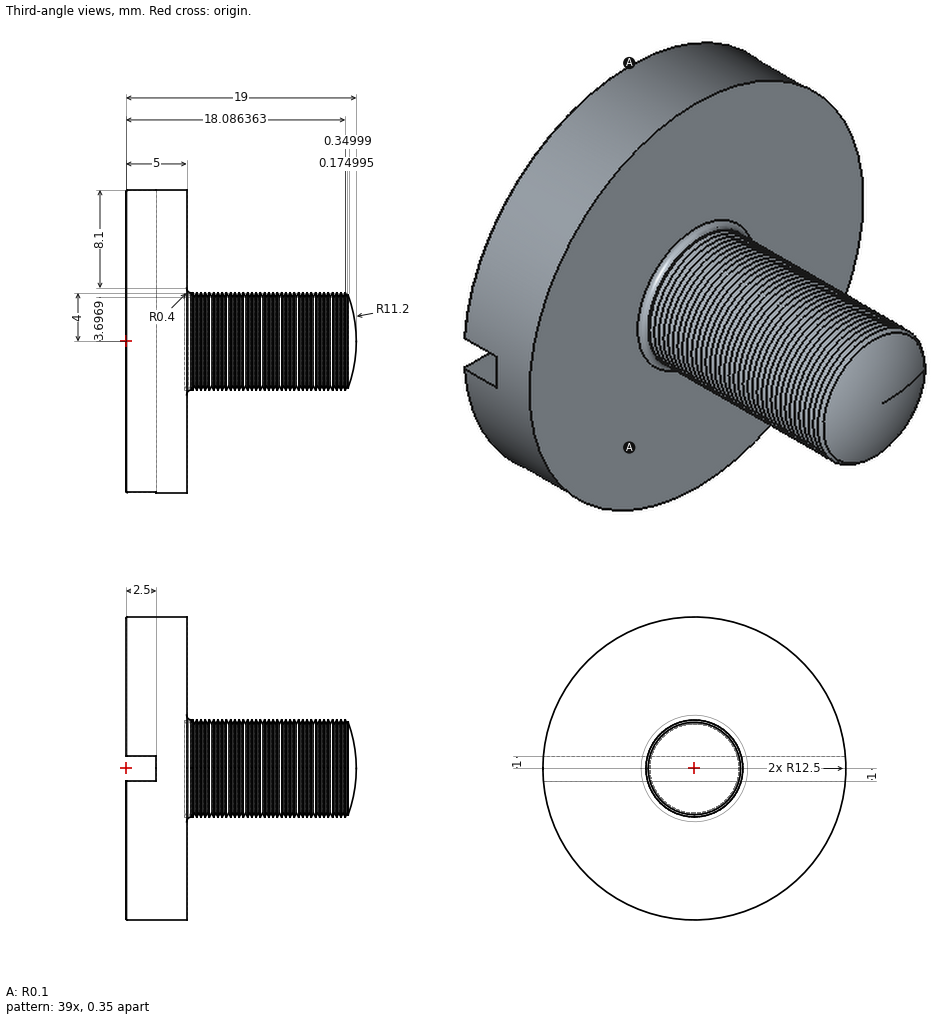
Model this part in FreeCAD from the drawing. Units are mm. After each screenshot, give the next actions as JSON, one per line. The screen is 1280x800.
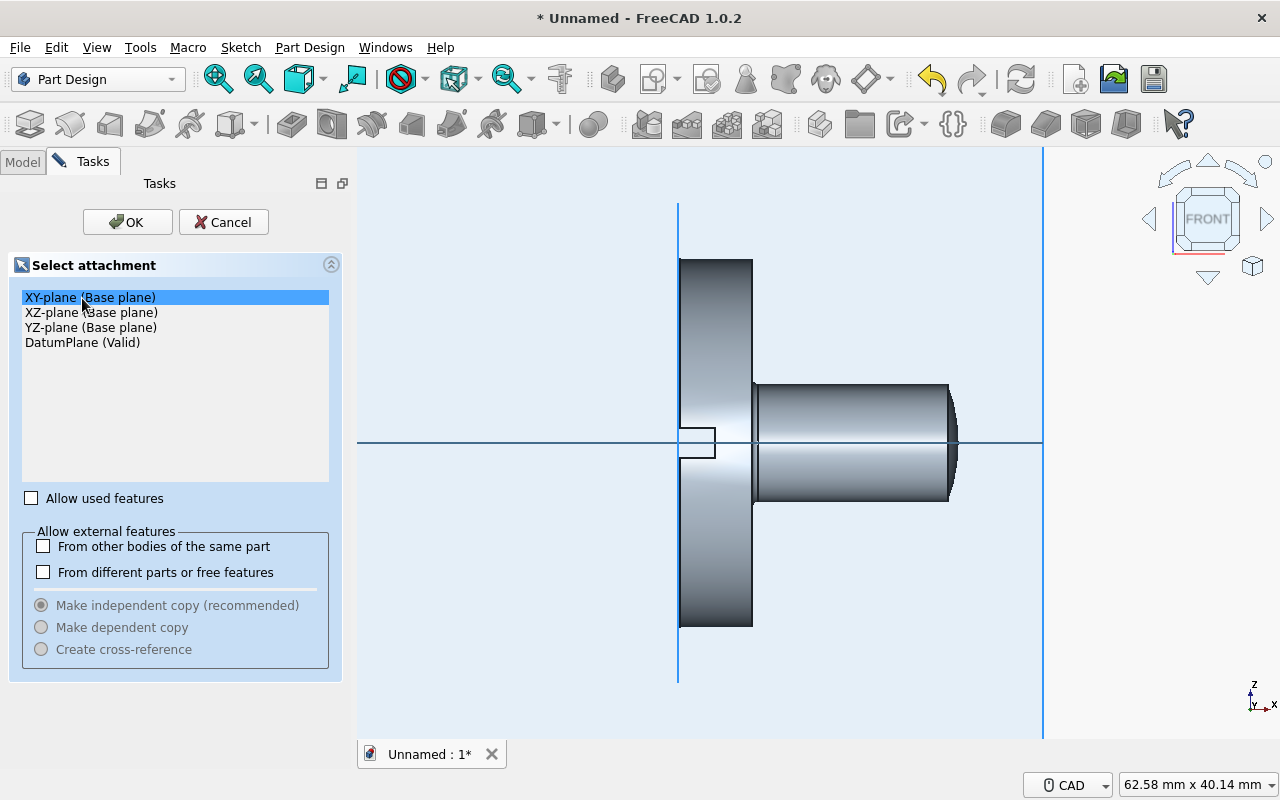
{"action": "left_click", "coordinate": [128, 222]}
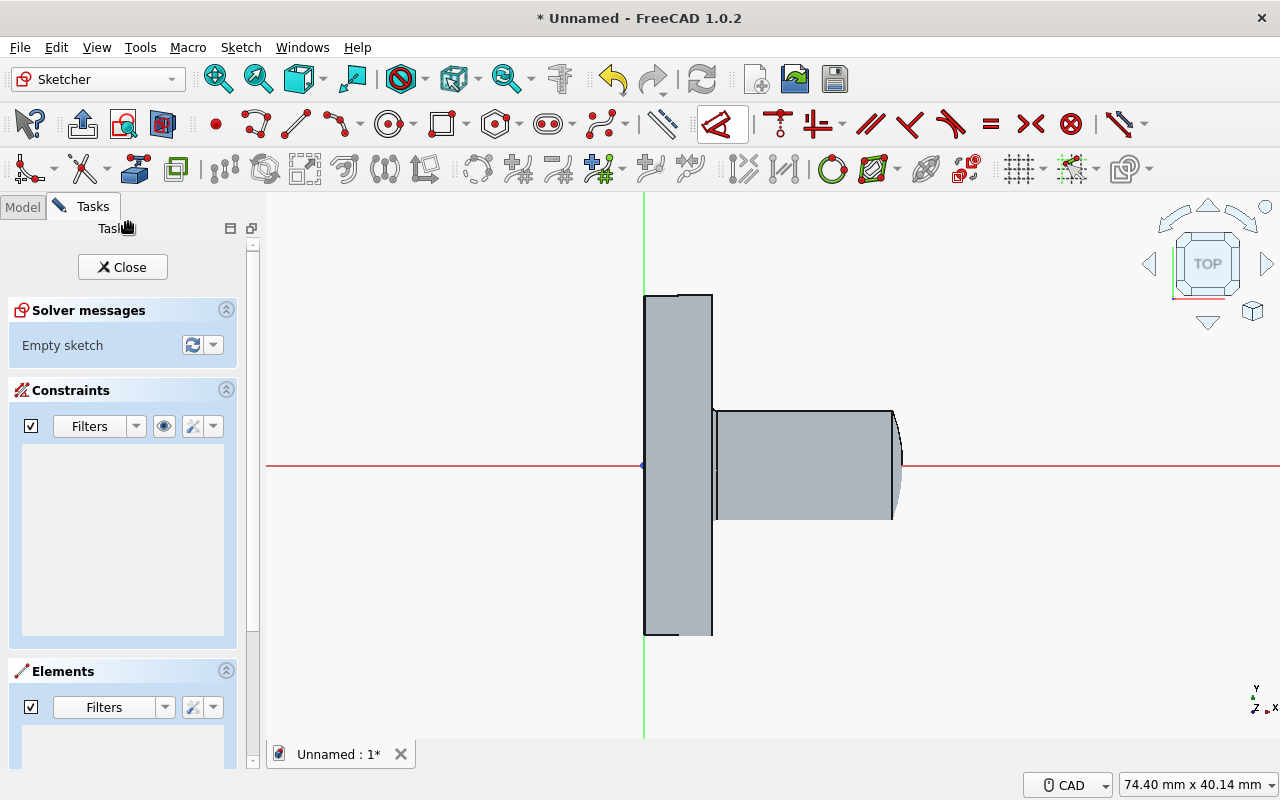
{"action": "left_click", "coordinate": [164, 124]}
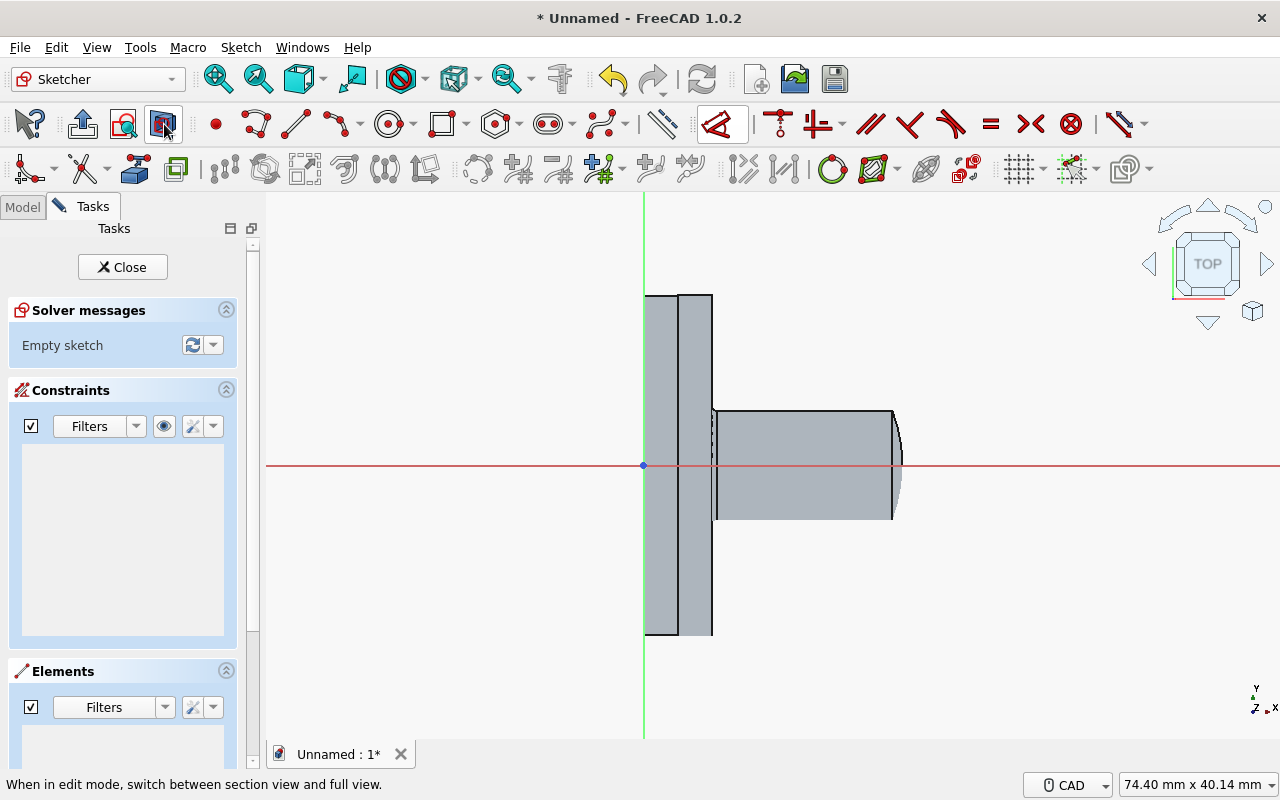
{"action": "scroll", "coordinate": [902, 410], "scroll_direction": "up", "scroll_amount": 15}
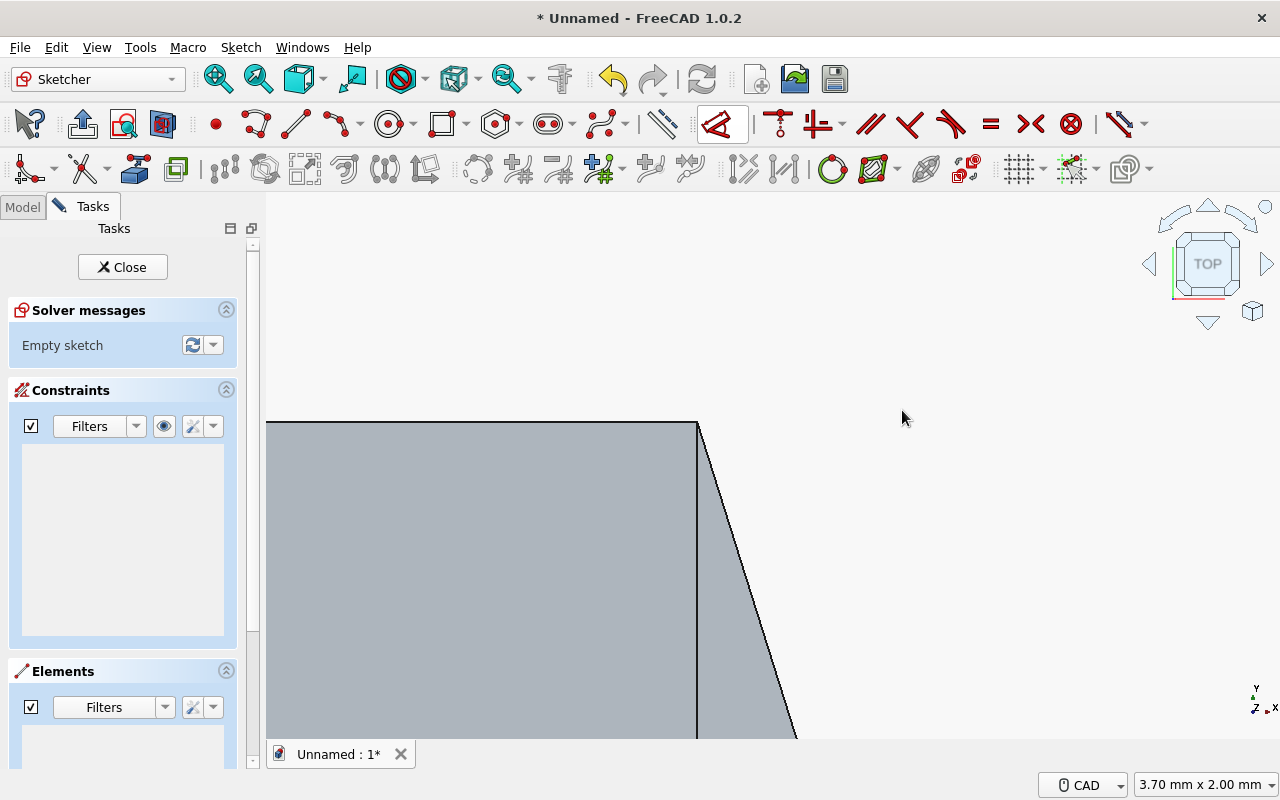
{"action": "scroll", "coordinate": [695, 463], "scroll_direction": "up", "scroll_amount": 7}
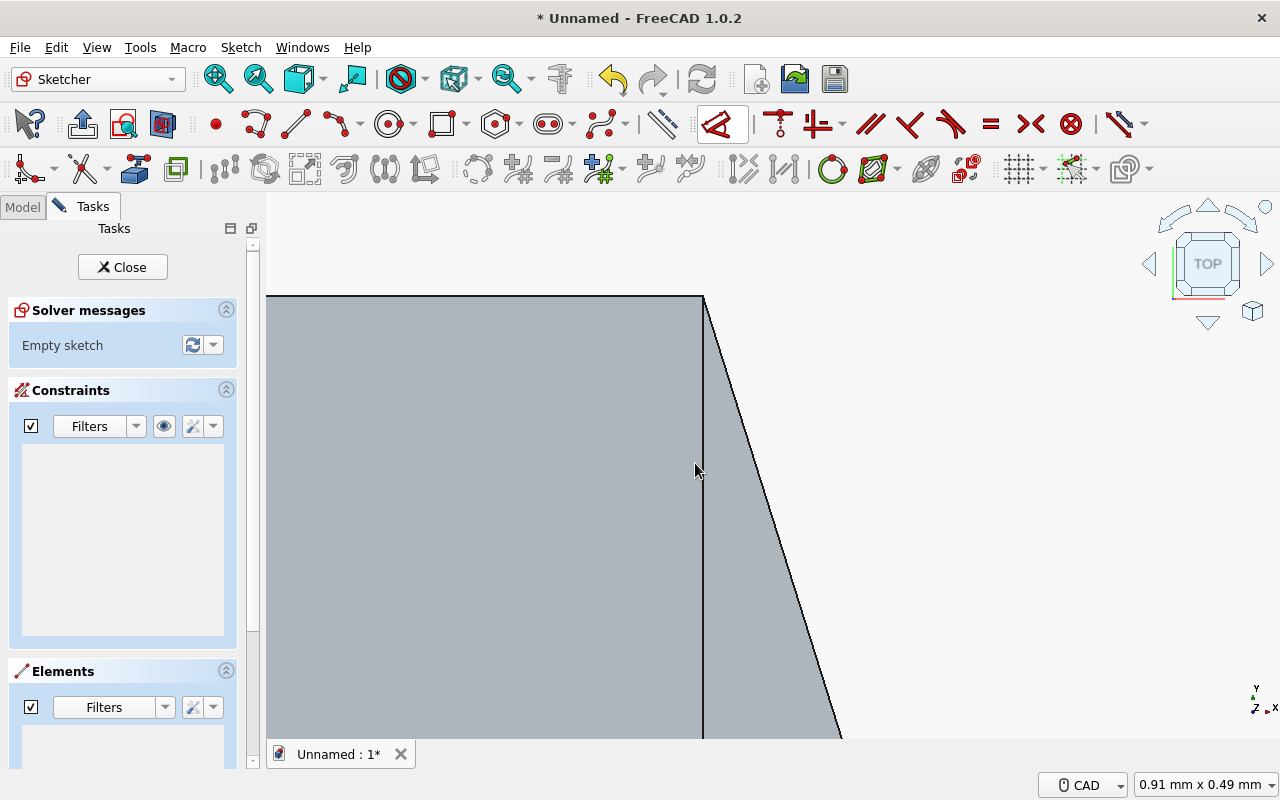
{"action": "left_click", "coordinate": [256, 124]}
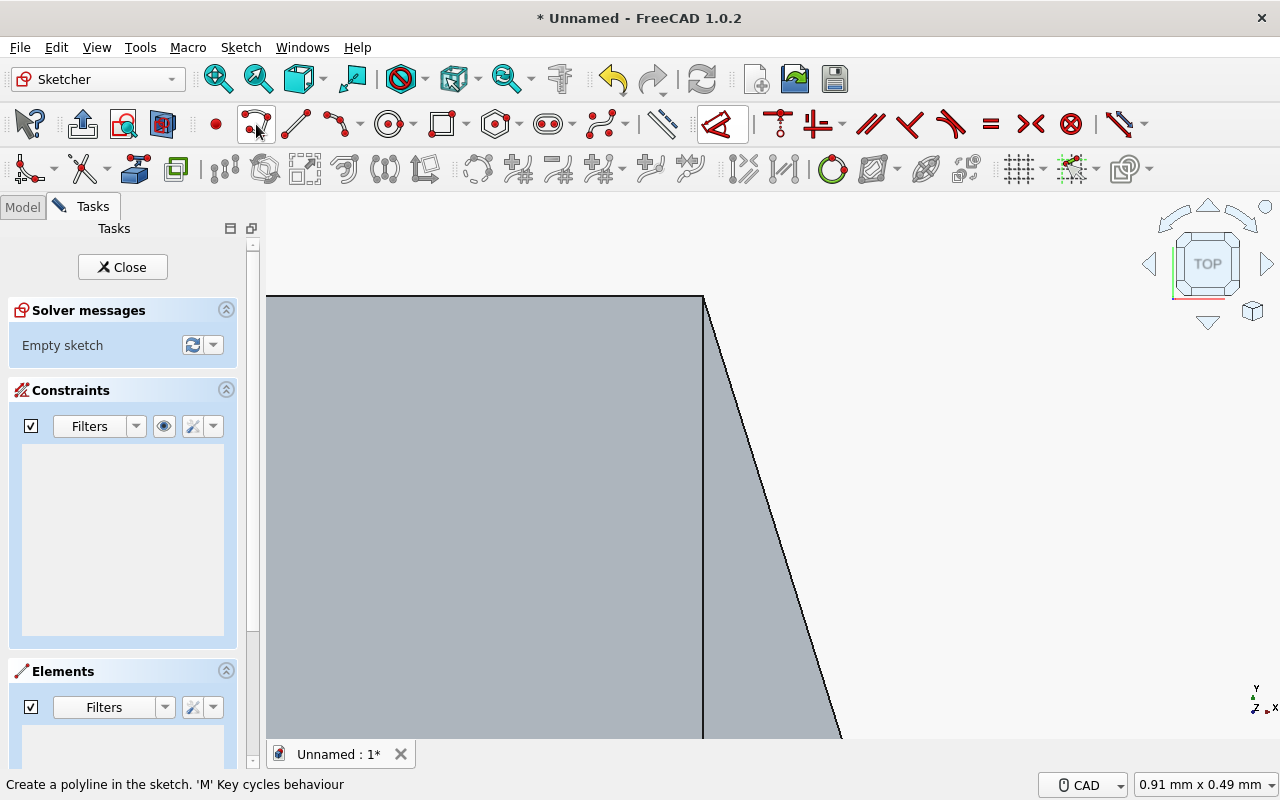
{"action": "left_click", "coordinate": [509, 296]}
{"action": "left_click", "coordinate": [703, 633]}
{"action": "left_click", "coordinate": [897, 296]}
{"action": "left_click", "coordinate": [509, 297]}
{"action": "key", "text": "Escape"}
{"action": "key", "text": "Escape"}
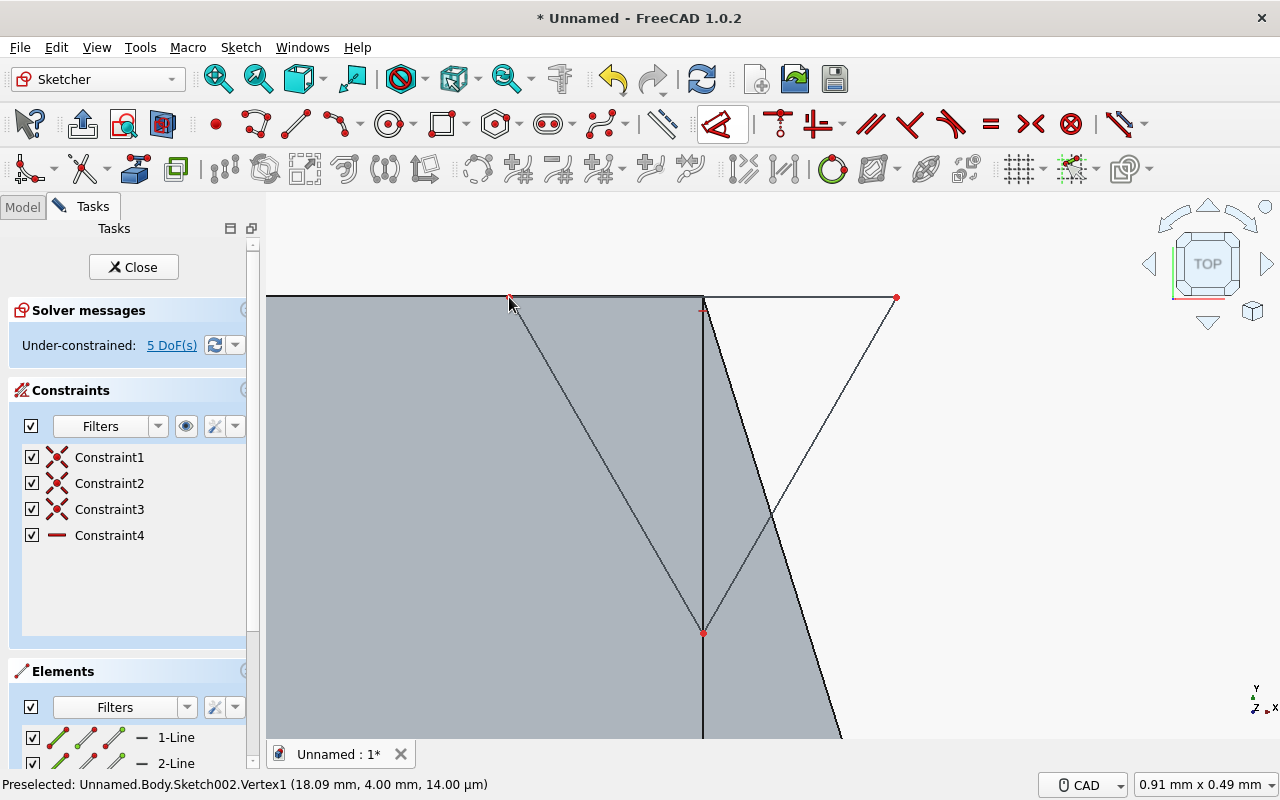
{"action": "left_click", "coordinate": [509, 297]}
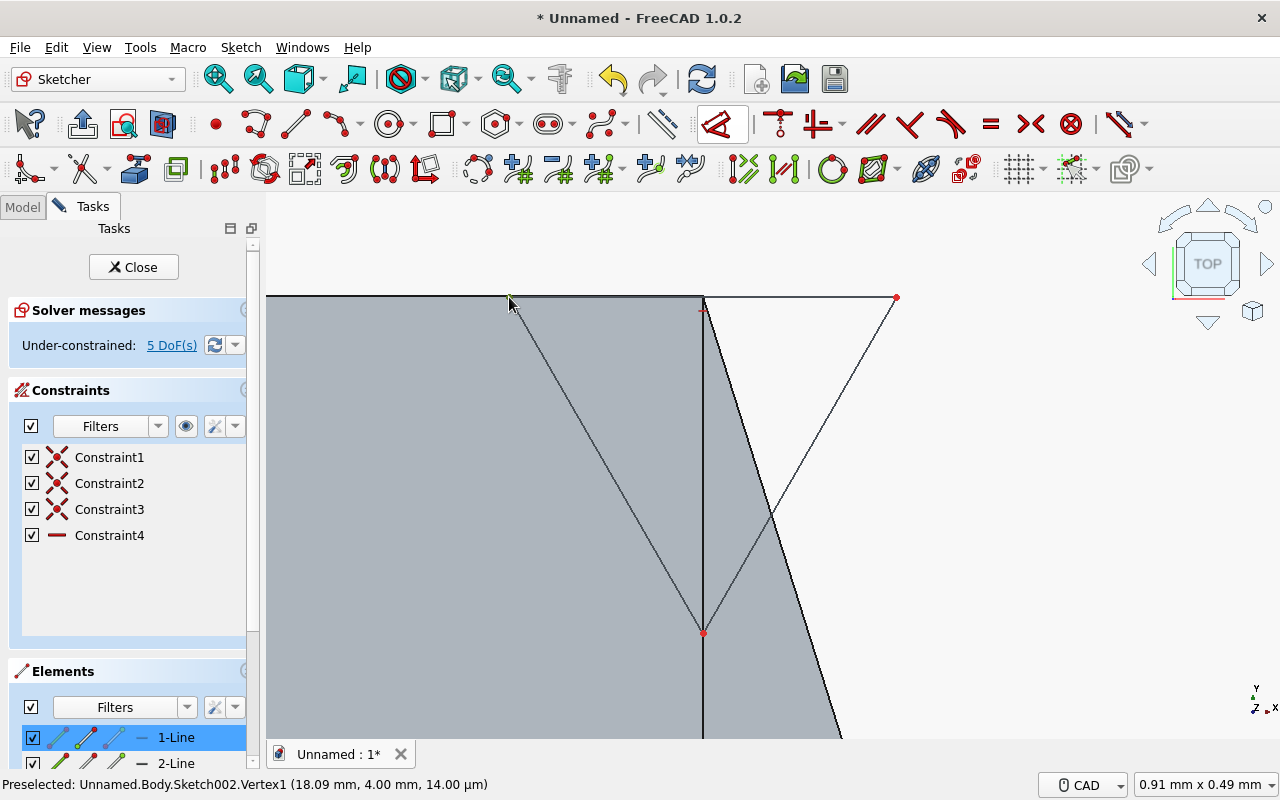
{"action": "key", "text": "i"}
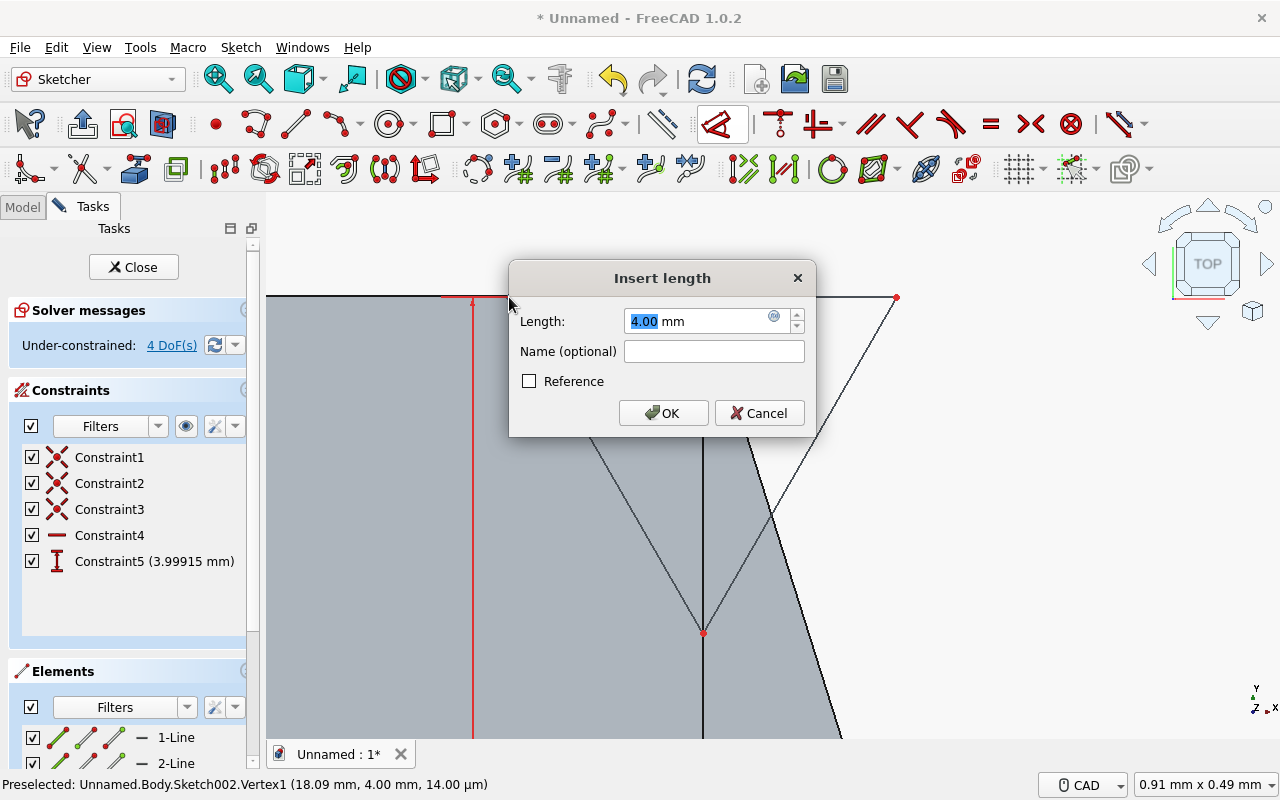
{"action": "type", "text": "4"}
{"action": "key", "text": "Return"}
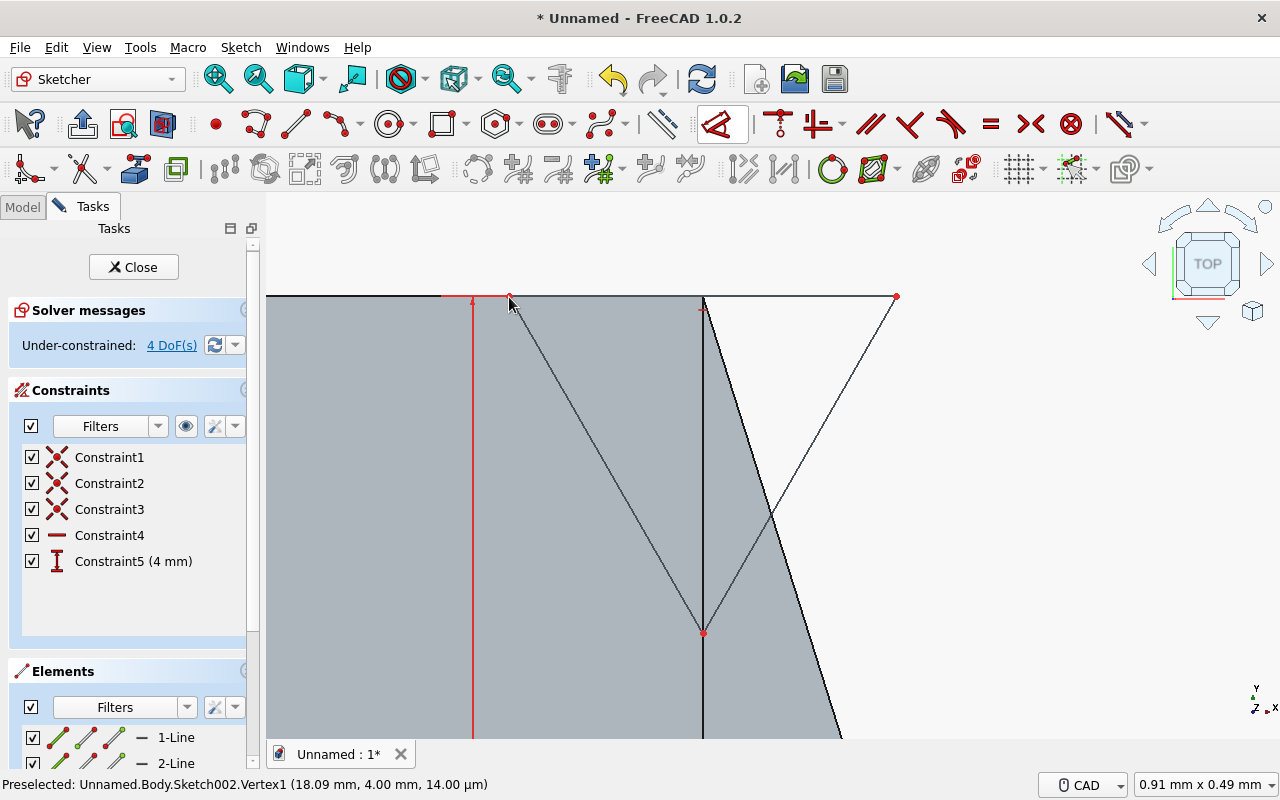
{"action": "left_click", "coordinate": [781, 296]}